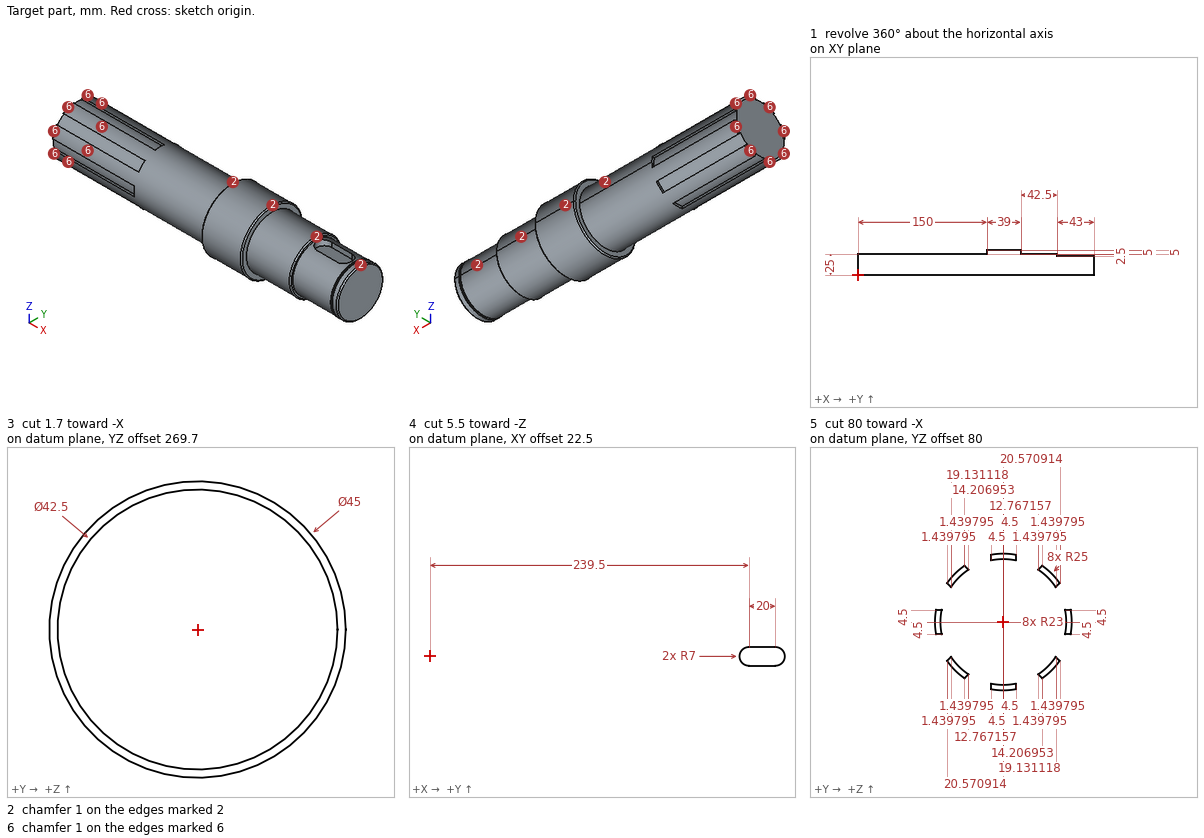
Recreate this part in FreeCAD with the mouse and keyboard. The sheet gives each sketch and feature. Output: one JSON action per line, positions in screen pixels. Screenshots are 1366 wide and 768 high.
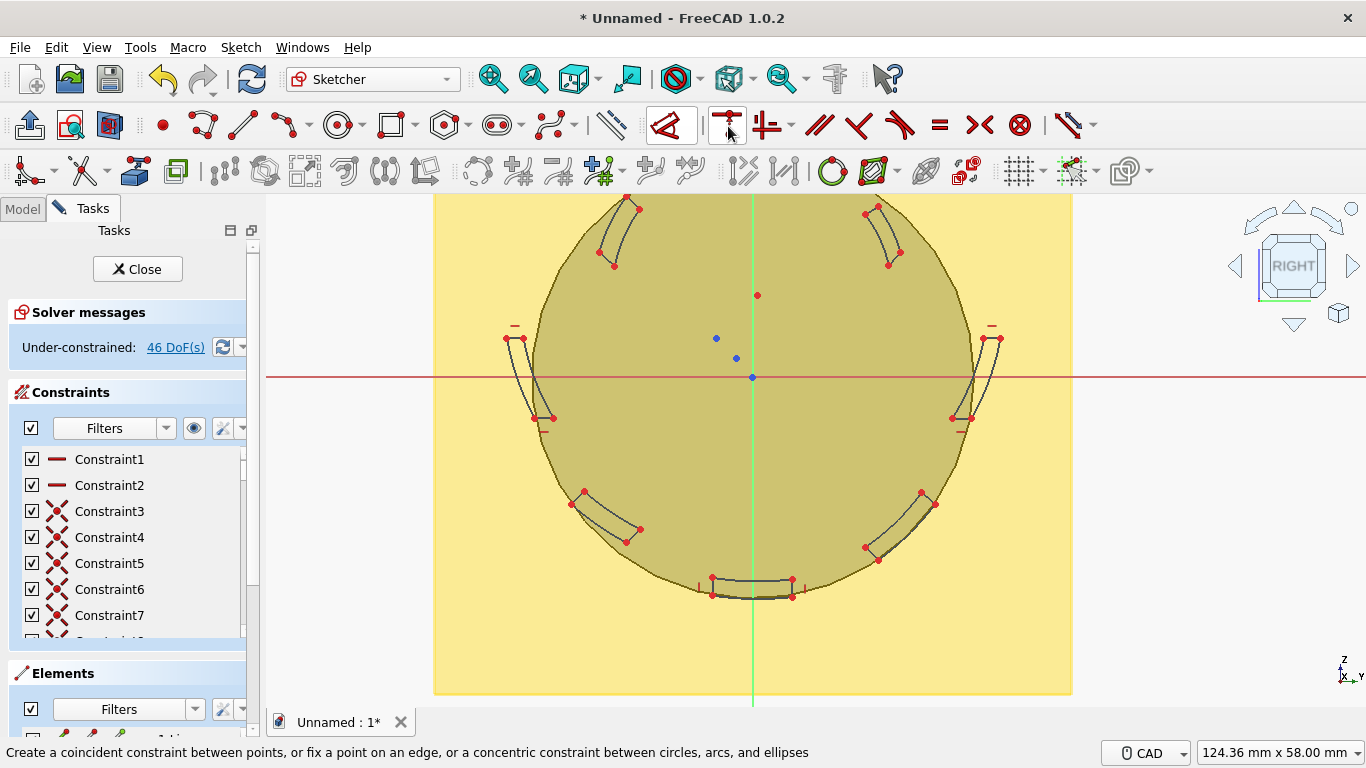
{"action": "left_click", "coordinate": [965, 396]}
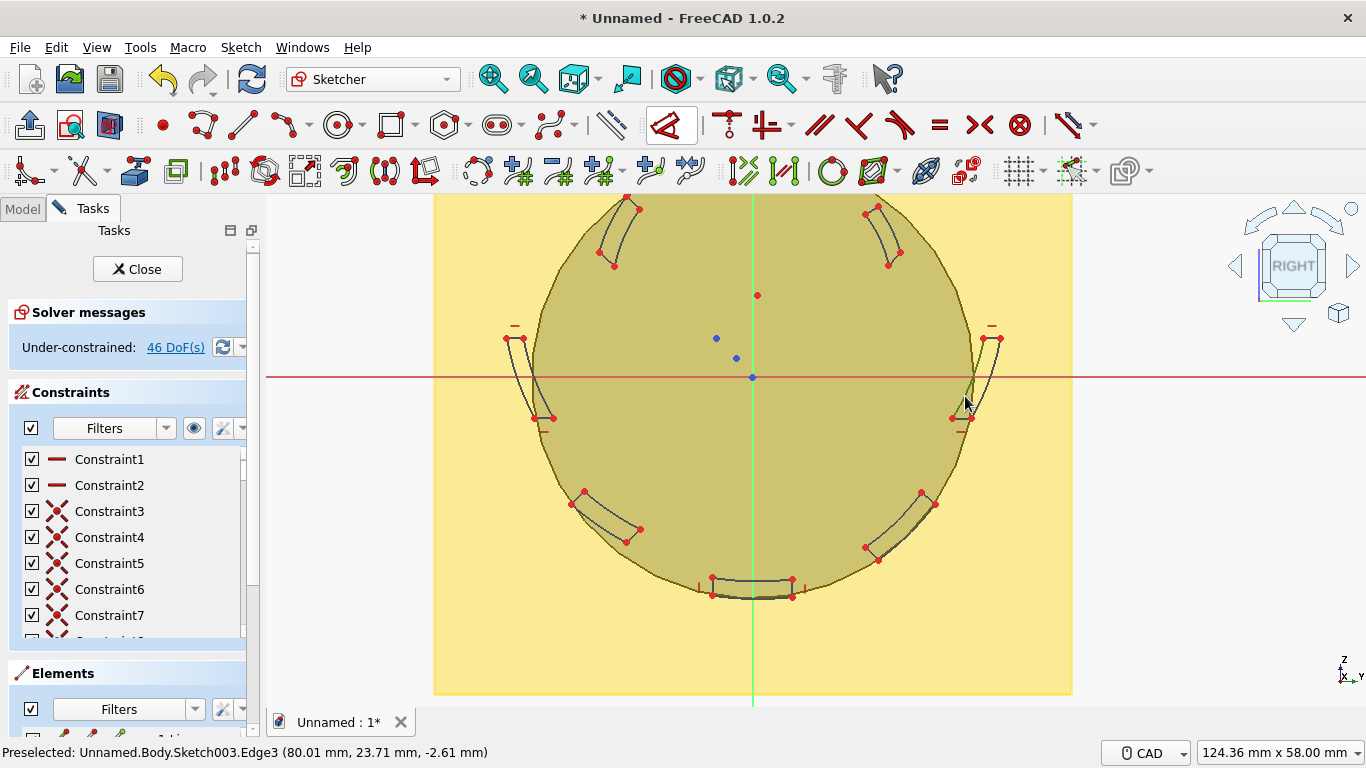
{"action": "left_click", "coordinate": [897, 545]}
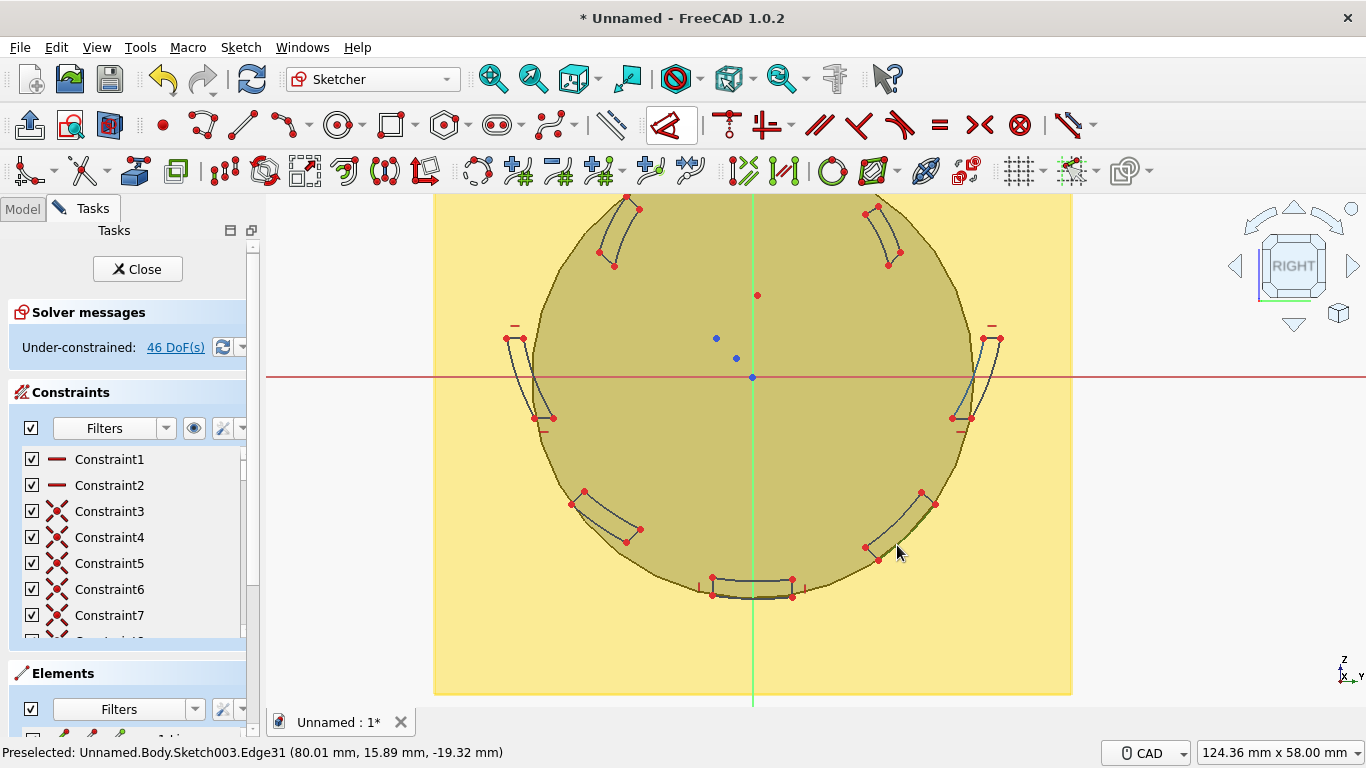
{"action": "left_click", "coordinate": [728, 126]}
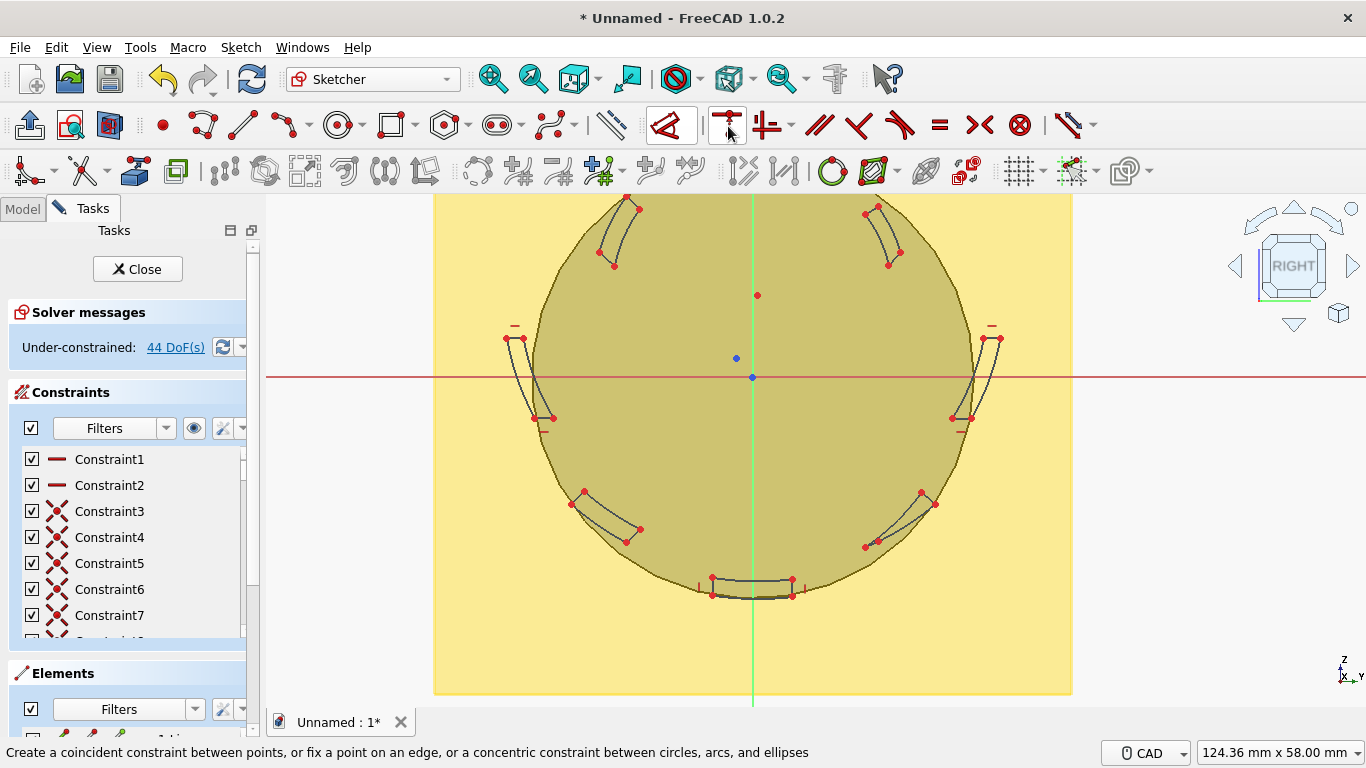
{"action": "left_click", "coordinate": [965, 396]}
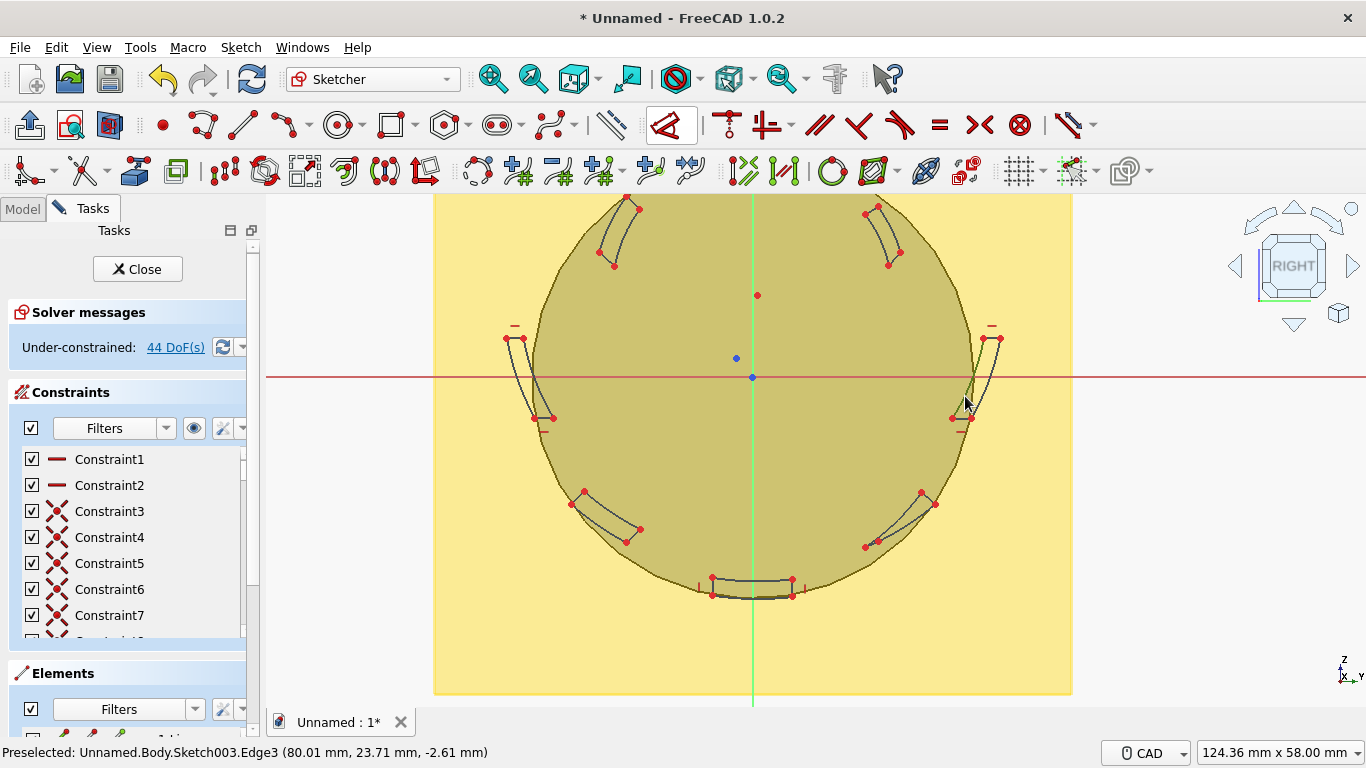
{"action": "left_click", "coordinate": [907, 511]}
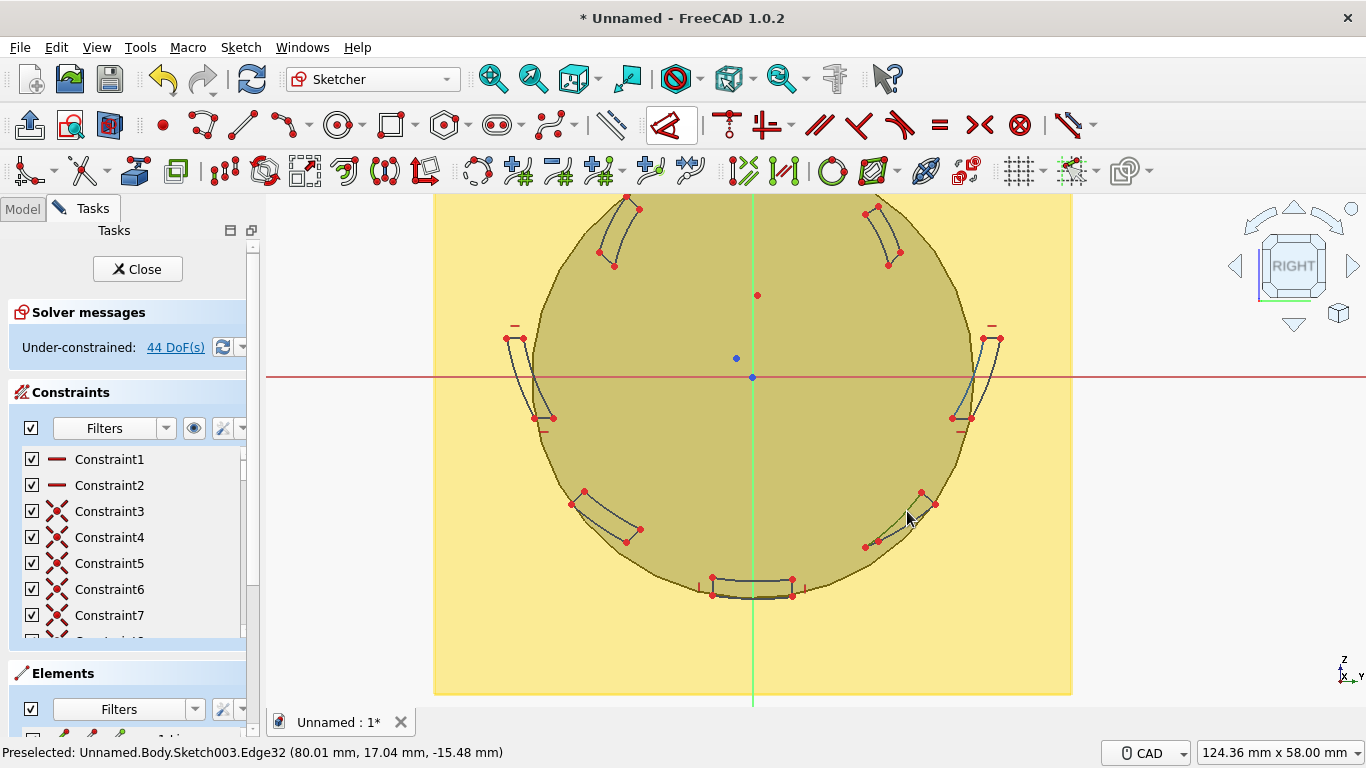
{"action": "left_click", "coordinate": [728, 126]}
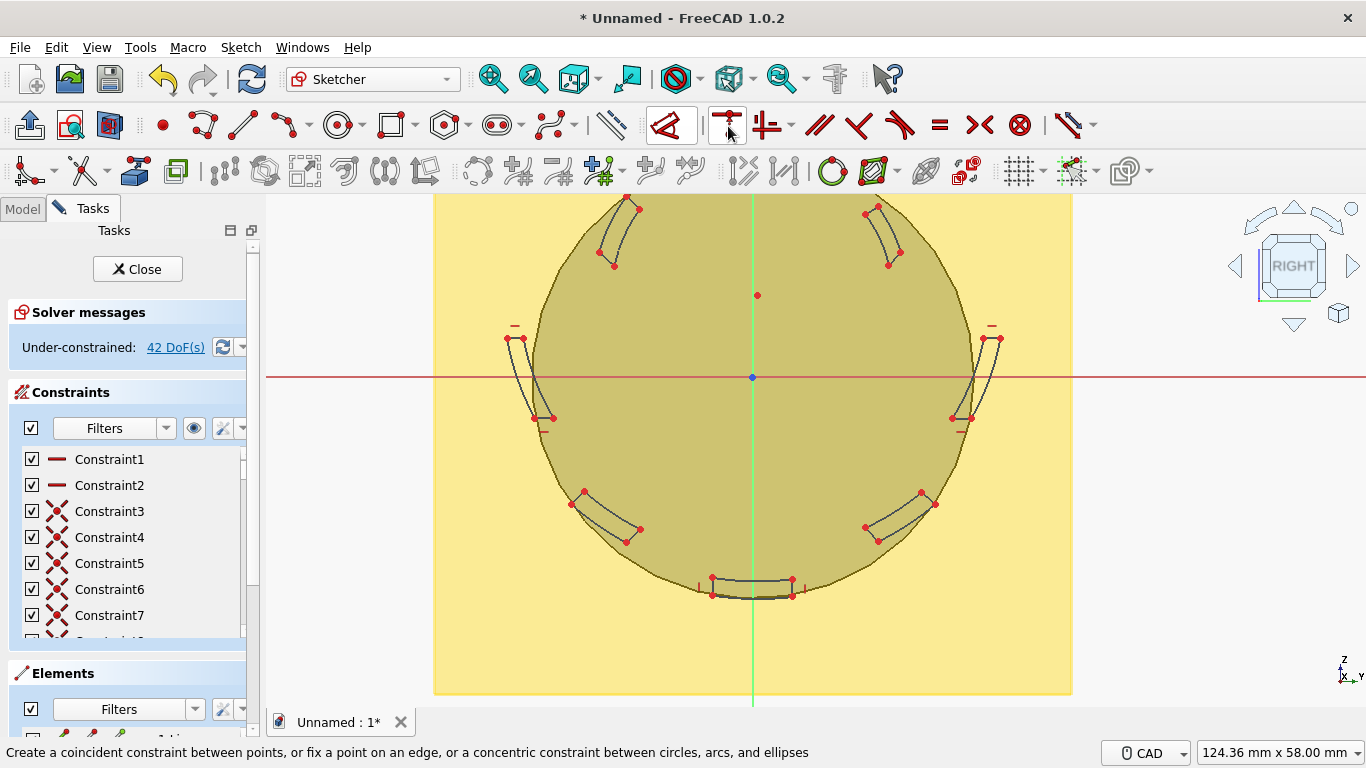
{"action": "left_click_drag", "start_coordinate": [743, 286], "coordinate": [768, 387]}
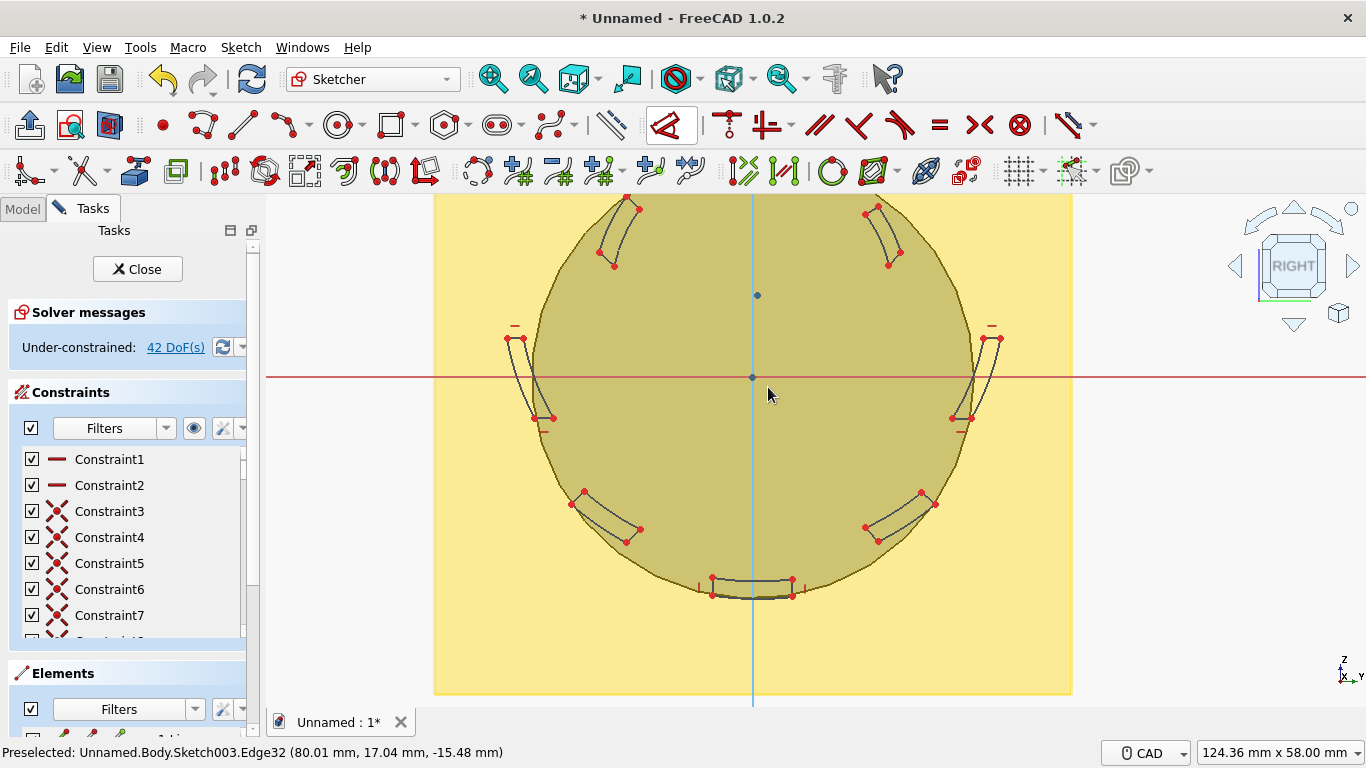
{"action": "left_click", "coordinate": [728, 126]}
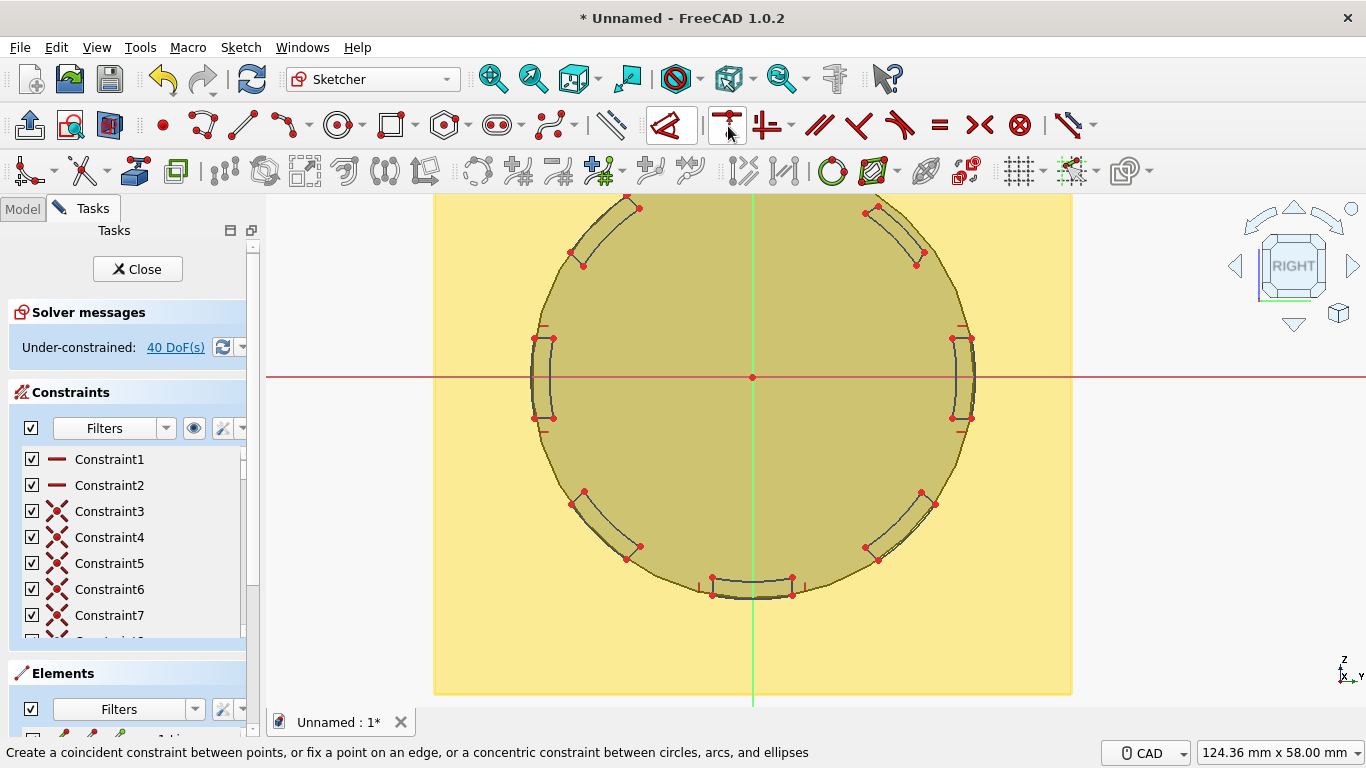
{"action": "left_click", "coordinate": [974, 395]}